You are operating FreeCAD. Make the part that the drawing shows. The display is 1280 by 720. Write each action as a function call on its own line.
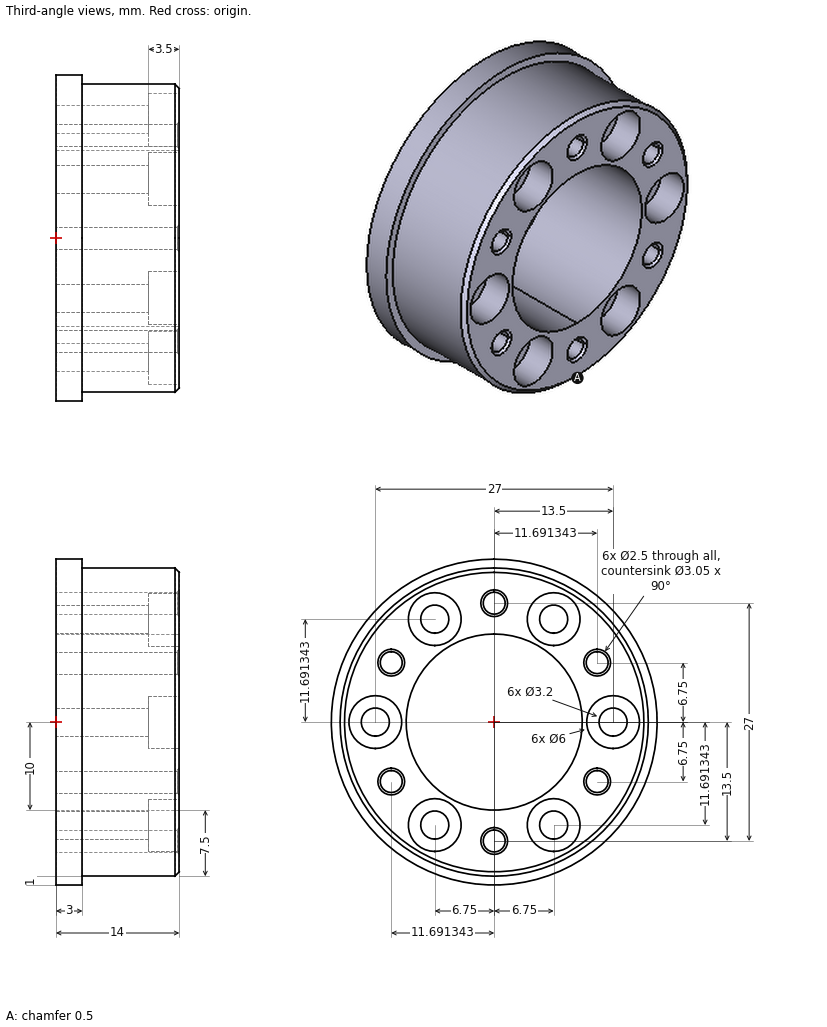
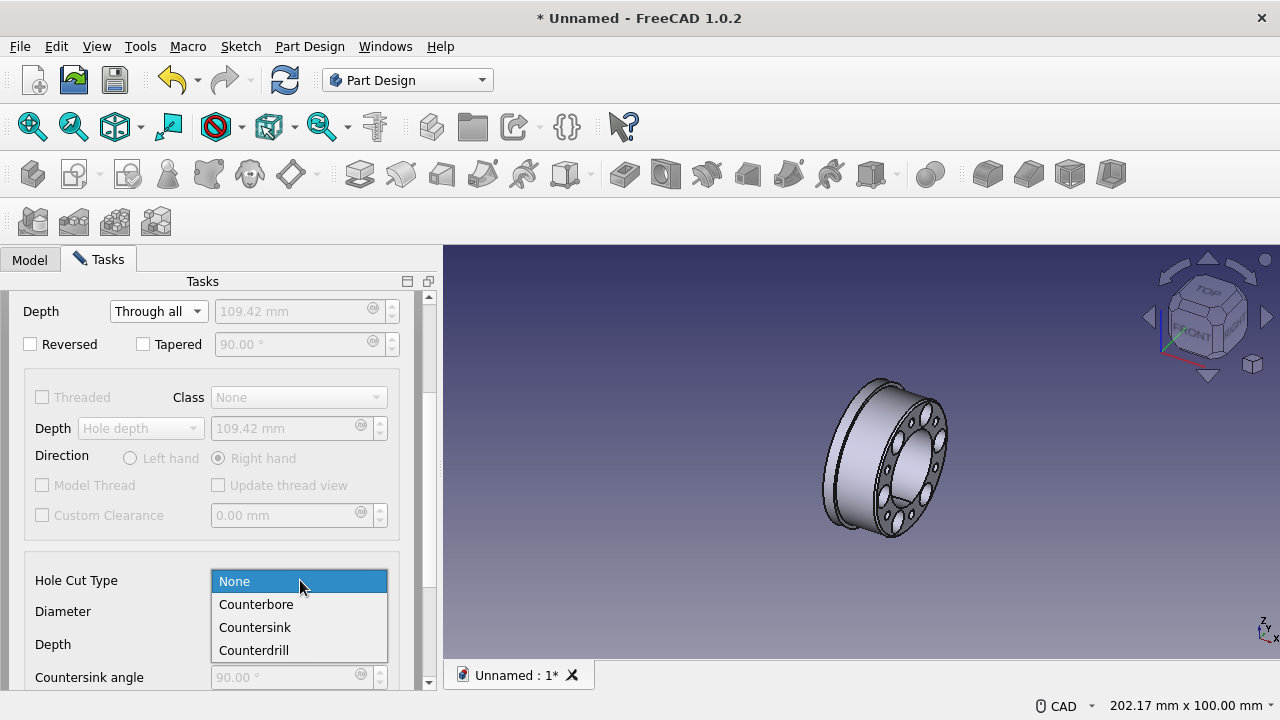
click(298, 628)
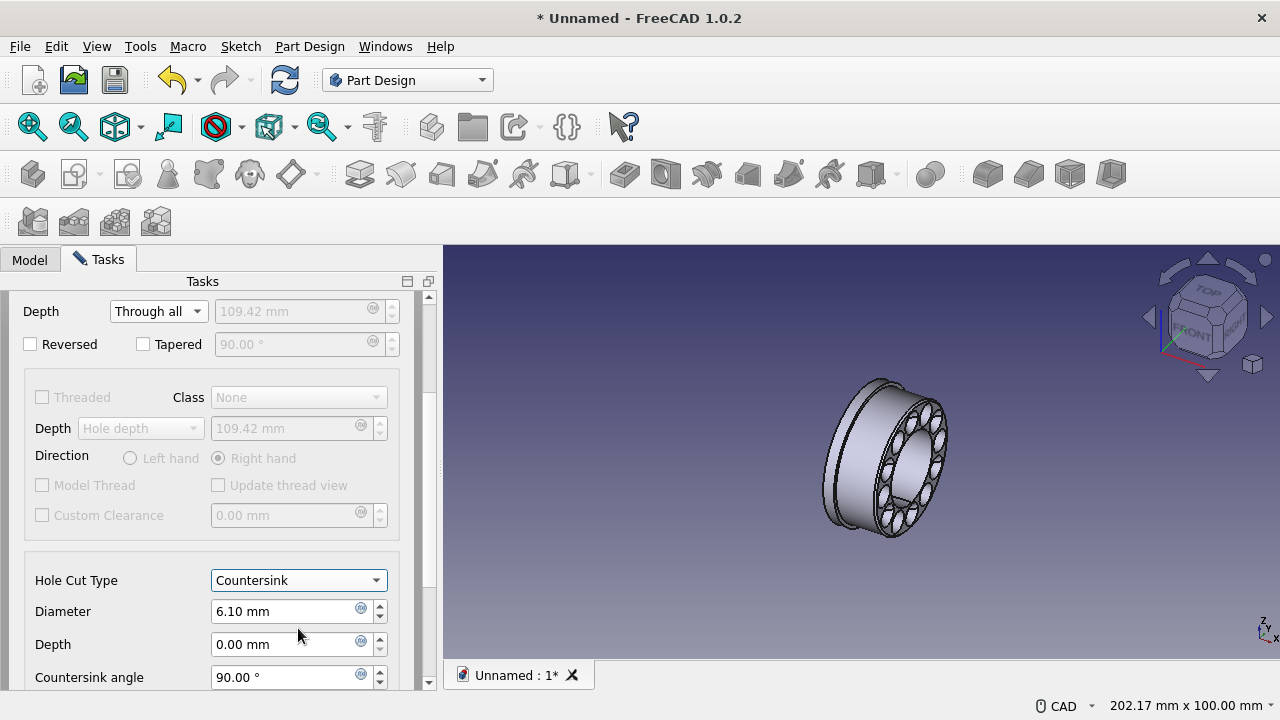
triple_click(292, 612)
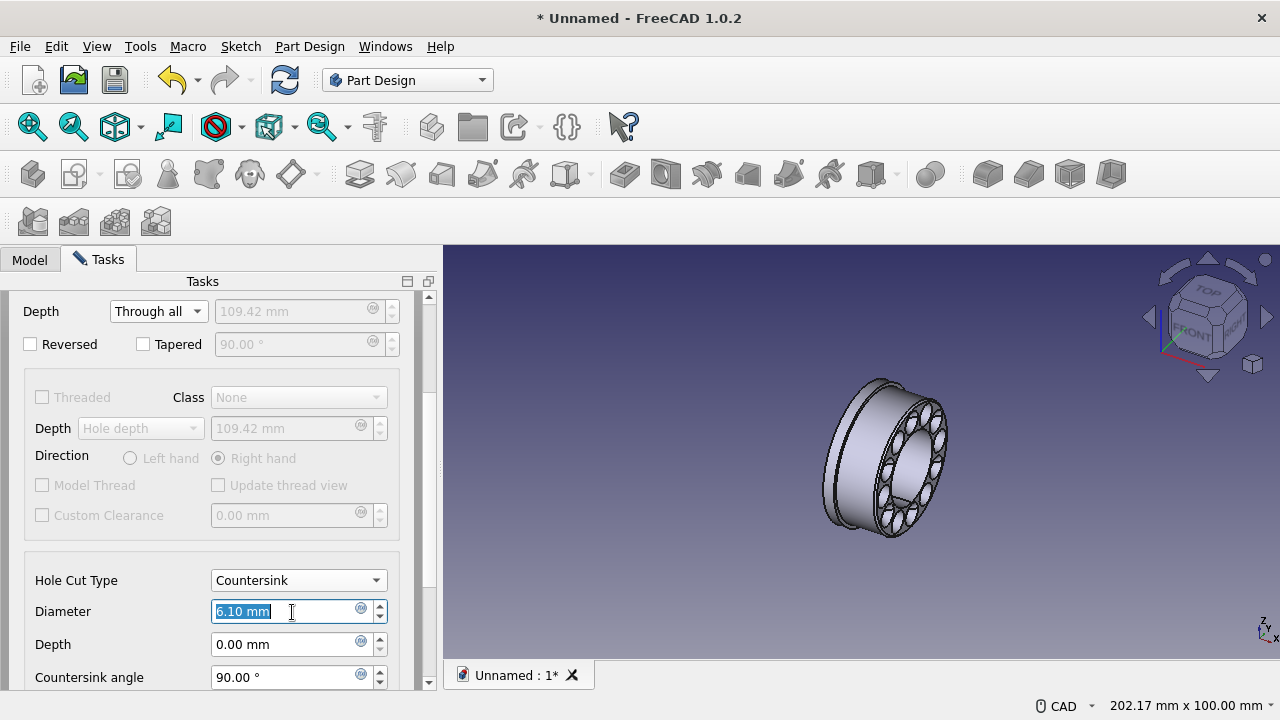
text(3.05)
key(Tab)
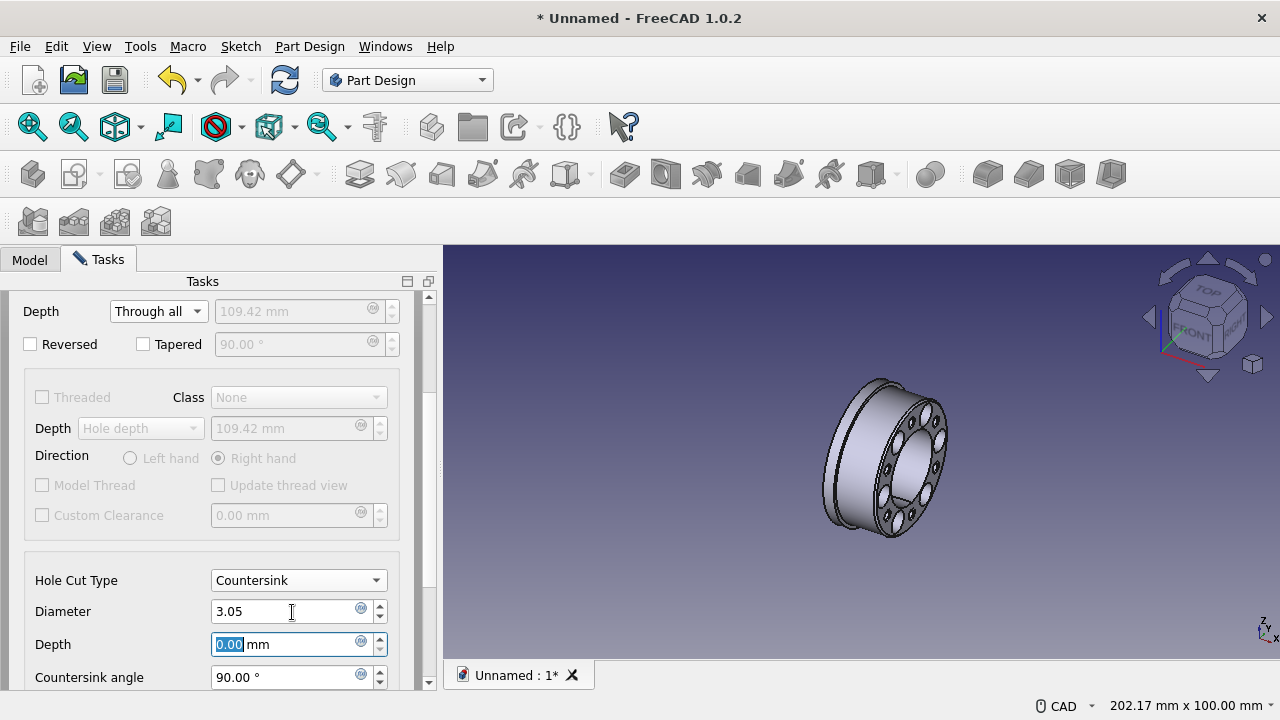
scroll(429, 490, up, 4)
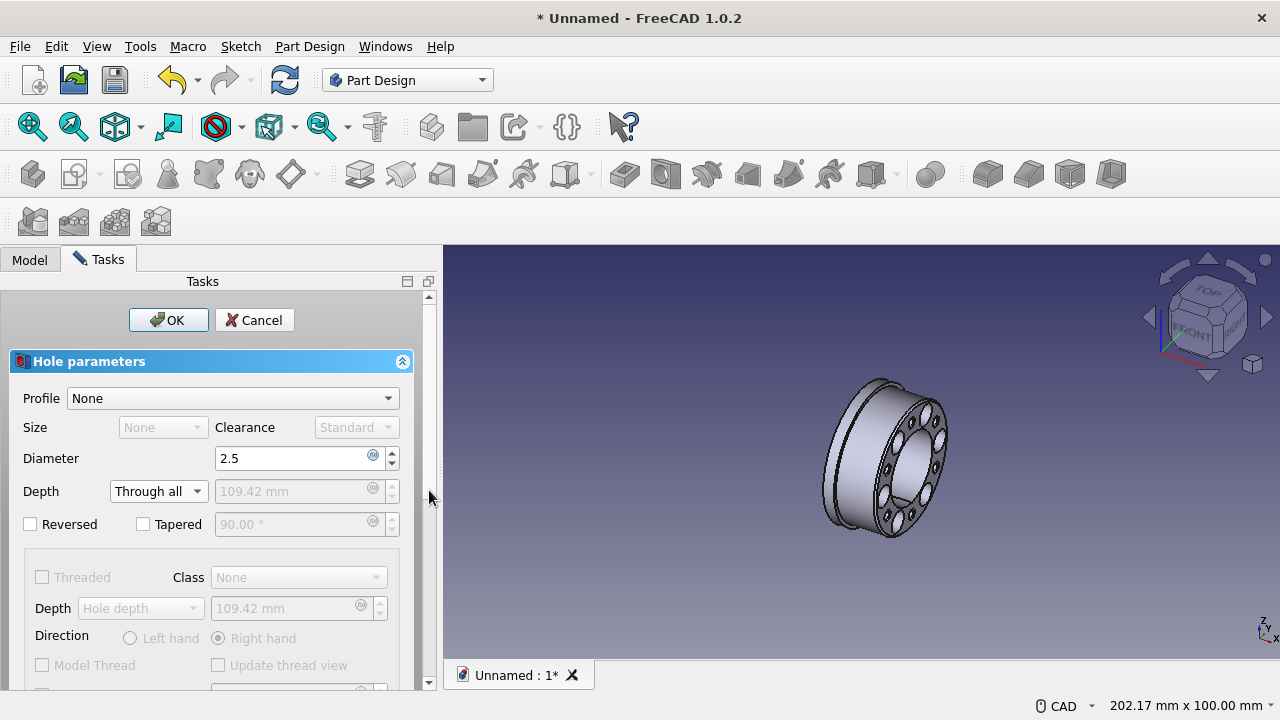
click(169, 320)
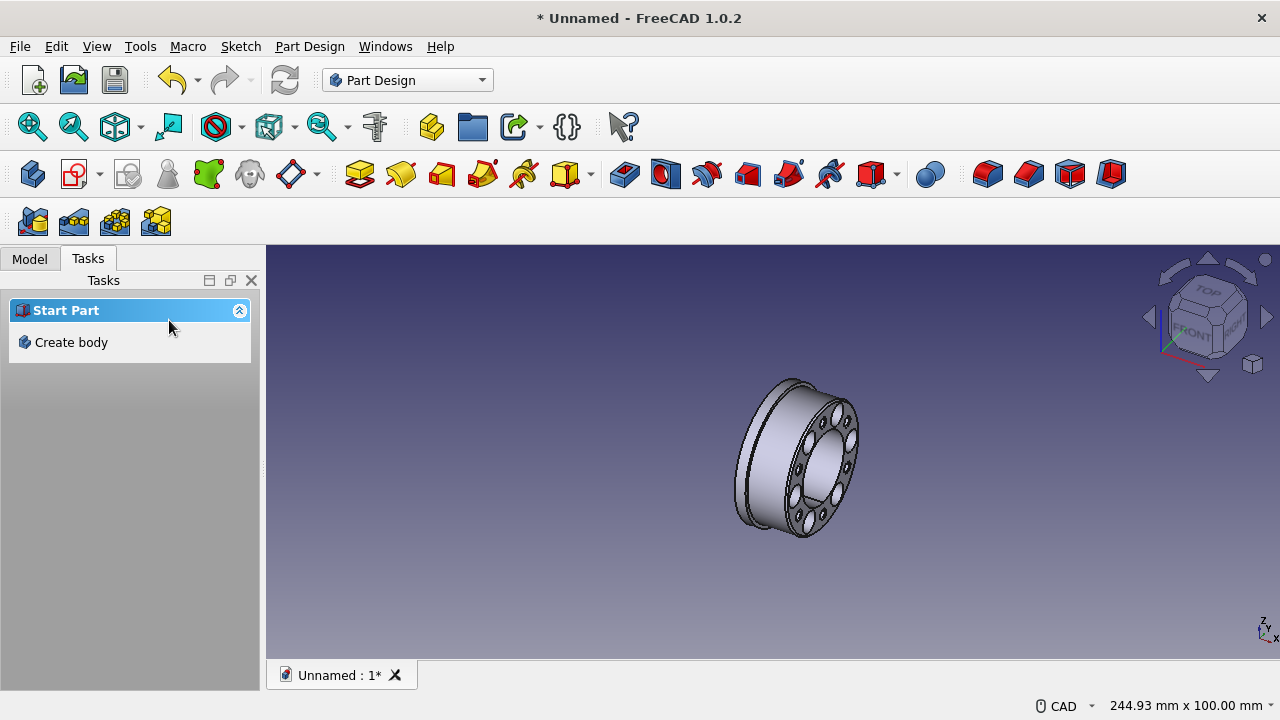
key(0)